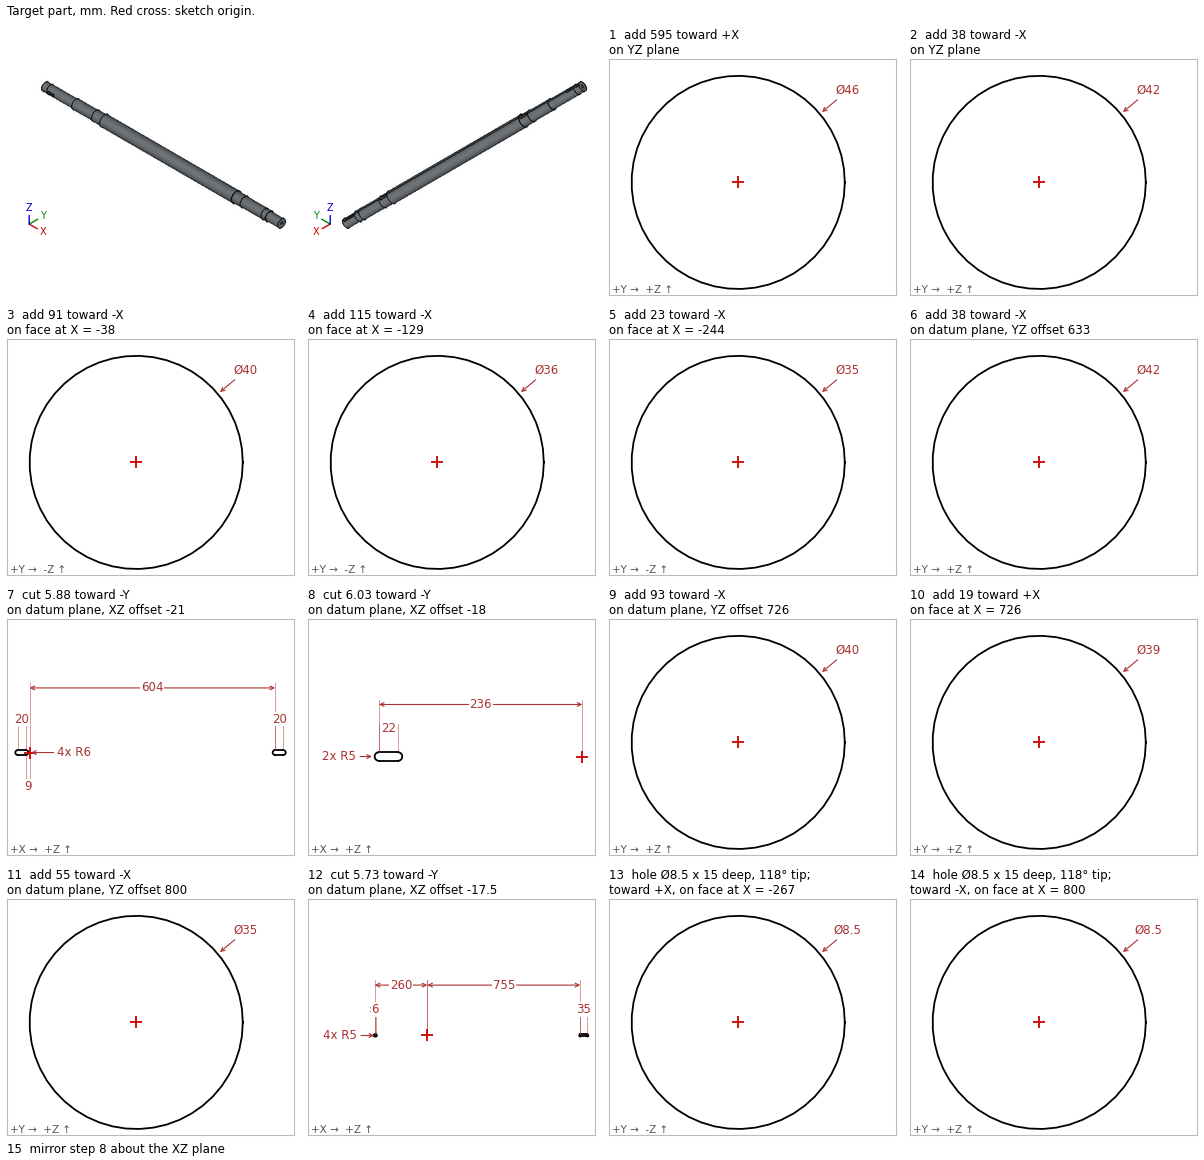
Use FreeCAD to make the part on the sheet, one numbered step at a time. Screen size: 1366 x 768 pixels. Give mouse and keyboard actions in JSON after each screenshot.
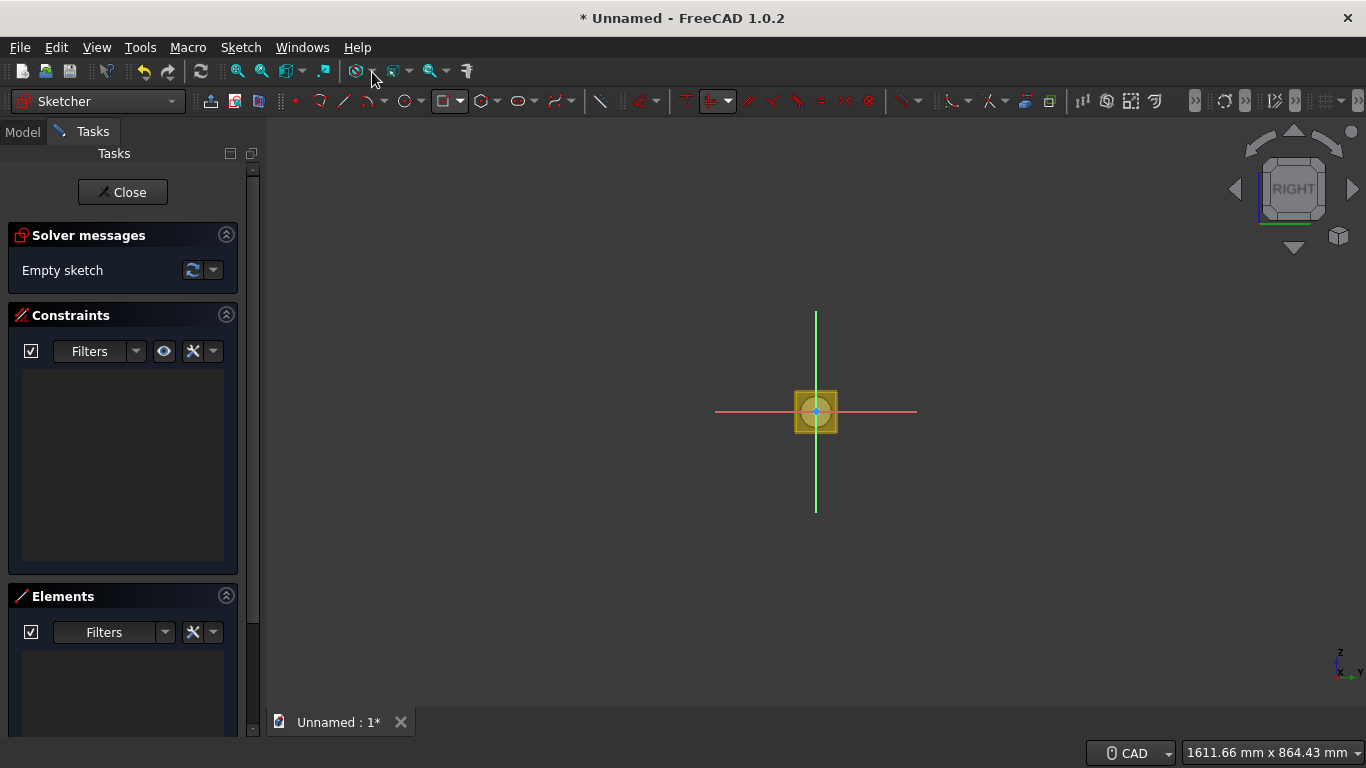
{"action": "scroll", "coordinate": [821, 412], "scroll_direction": "up", "scroll_amount": 13}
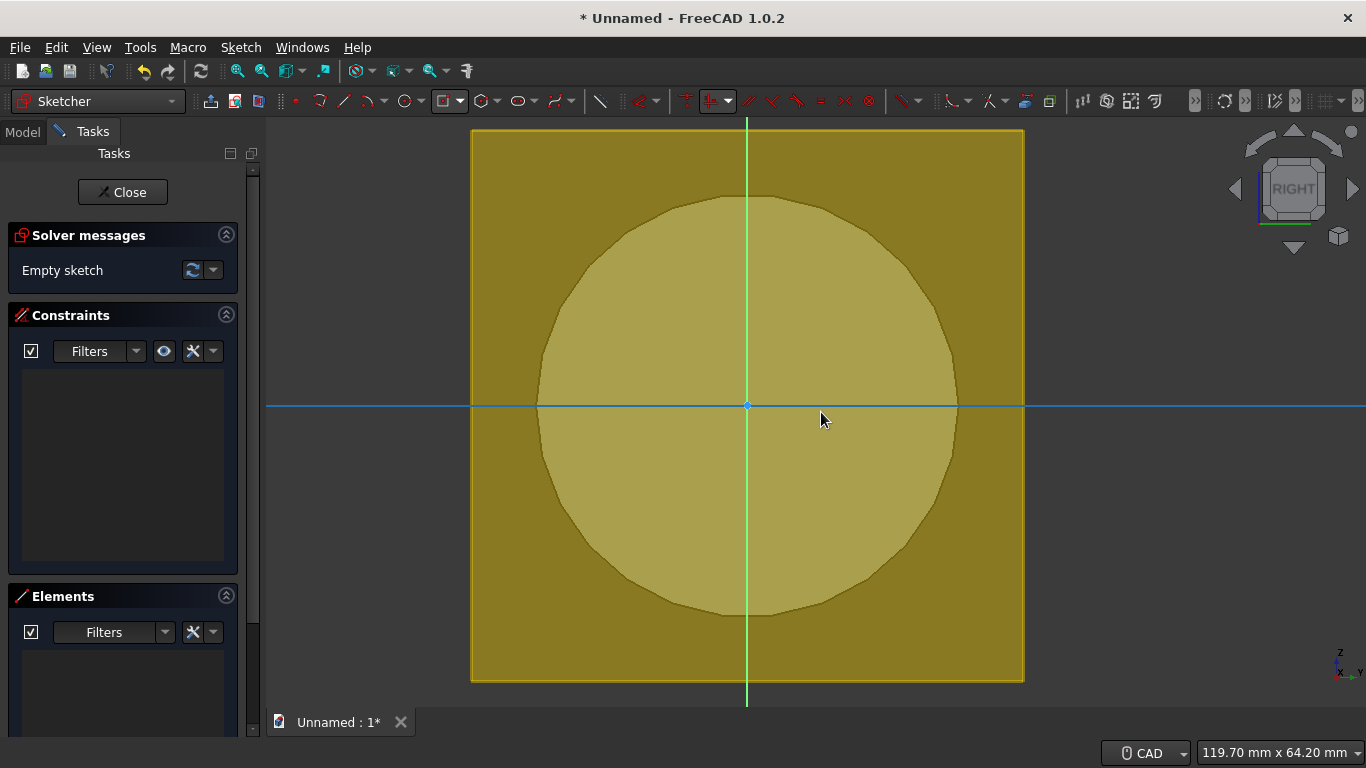
{"action": "key", "text": "g c"}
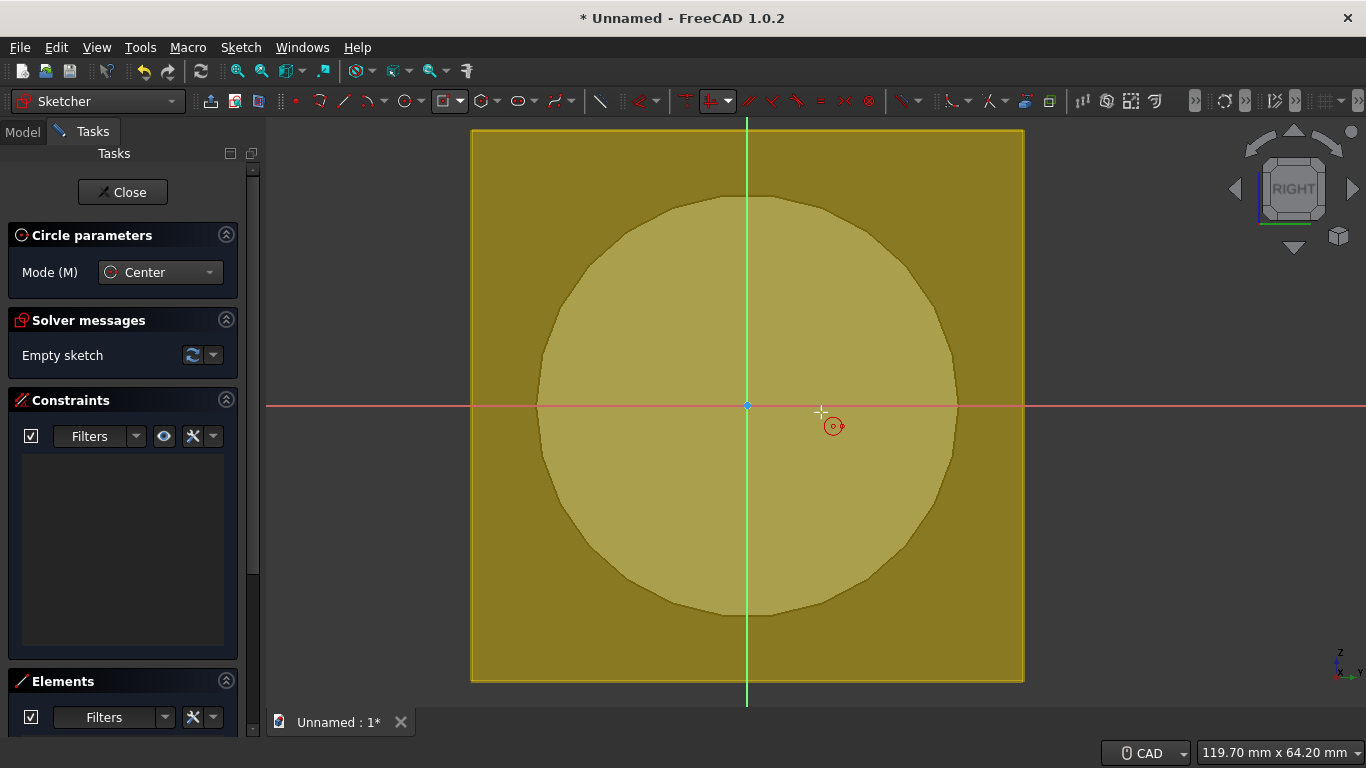
{"action": "left_click", "coordinate": [747, 406]}
{"action": "mouse_move", "coordinate": [884, 269]}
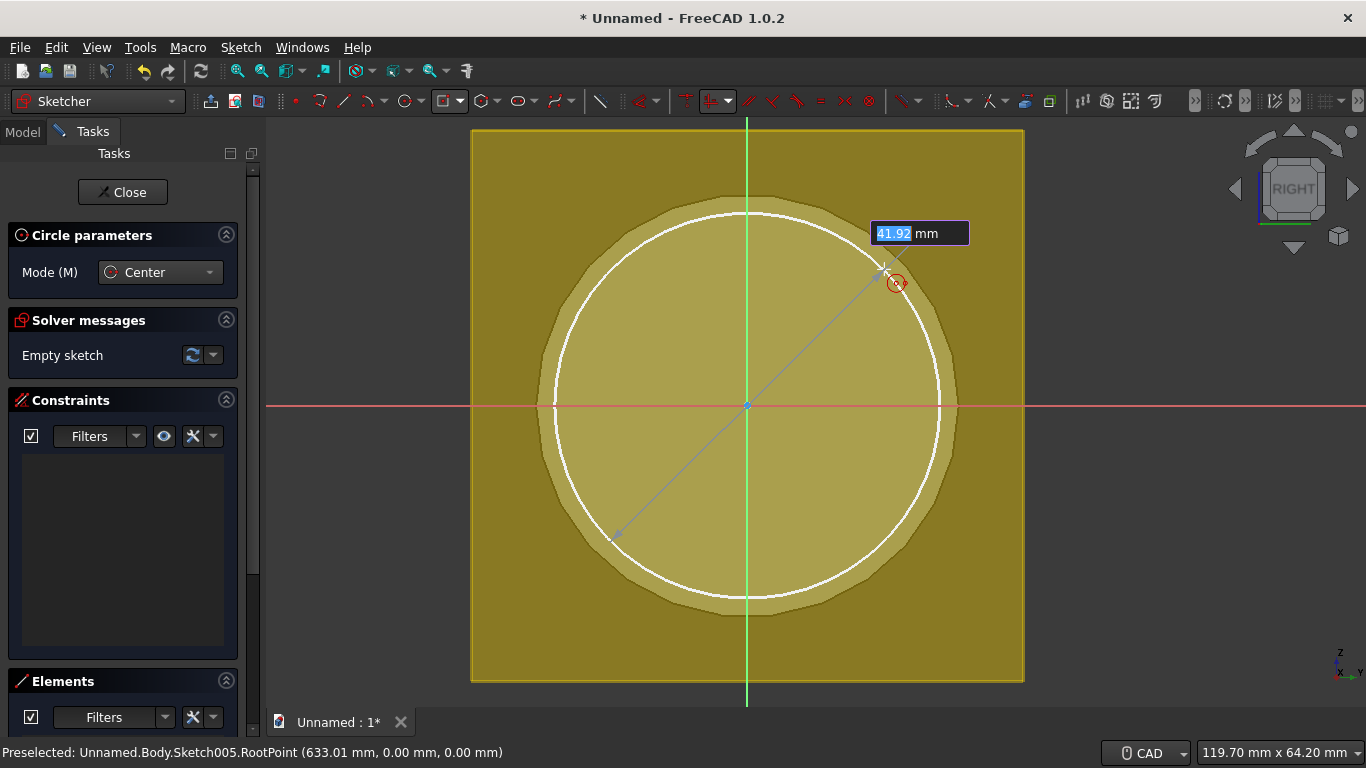
{"action": "type", "text": "42"}
{"action": "key", "text": "Return"}
{"action": "key", "text": "Escape"}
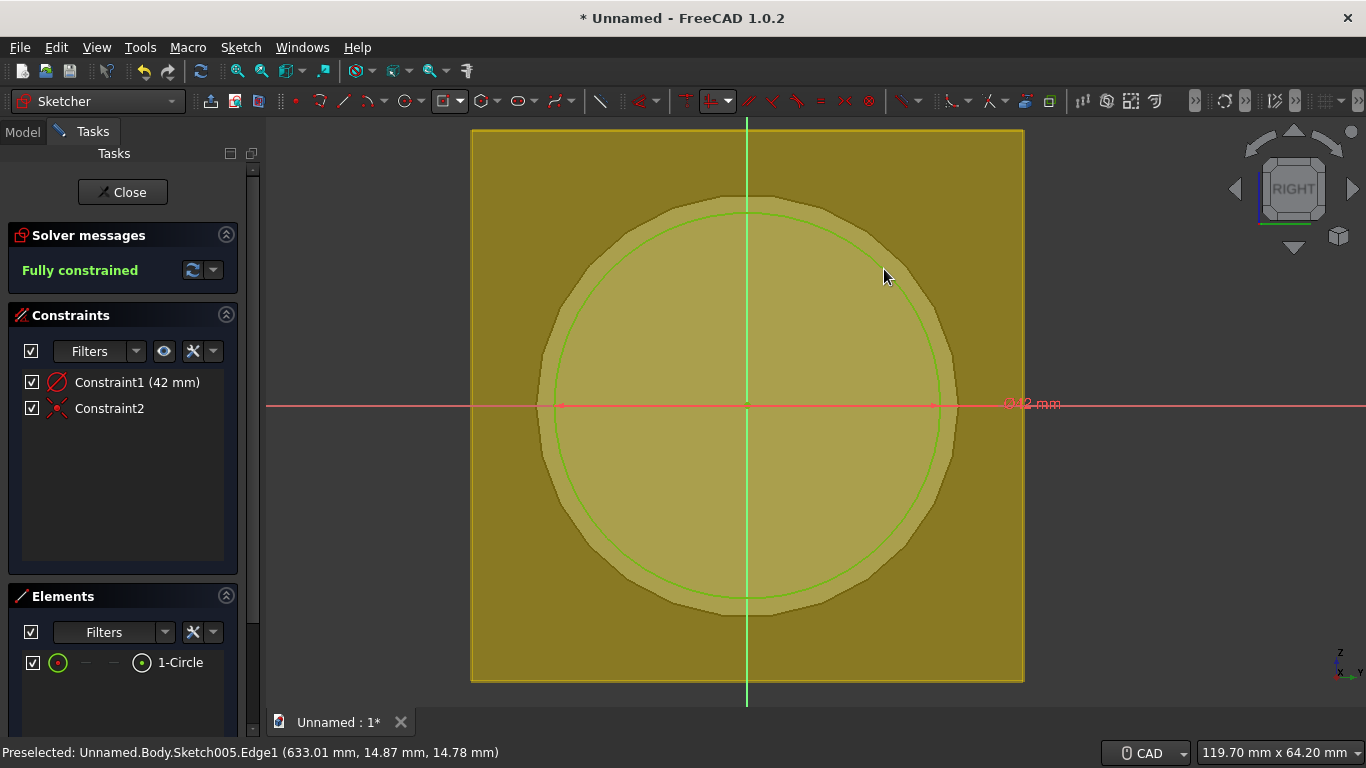
{"action": "left_click", "coordinate": [123, 192]}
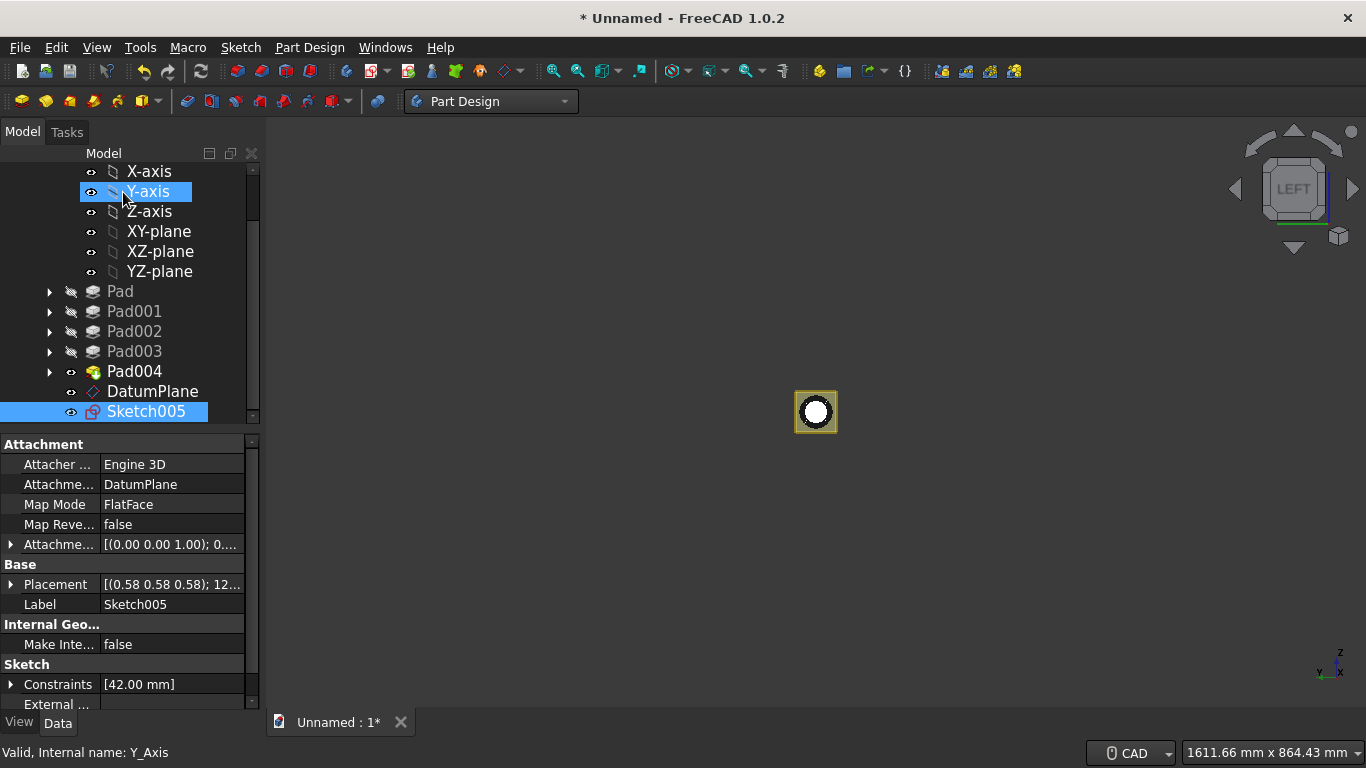
{"action": "left_click", "coordinate": [22, 102]}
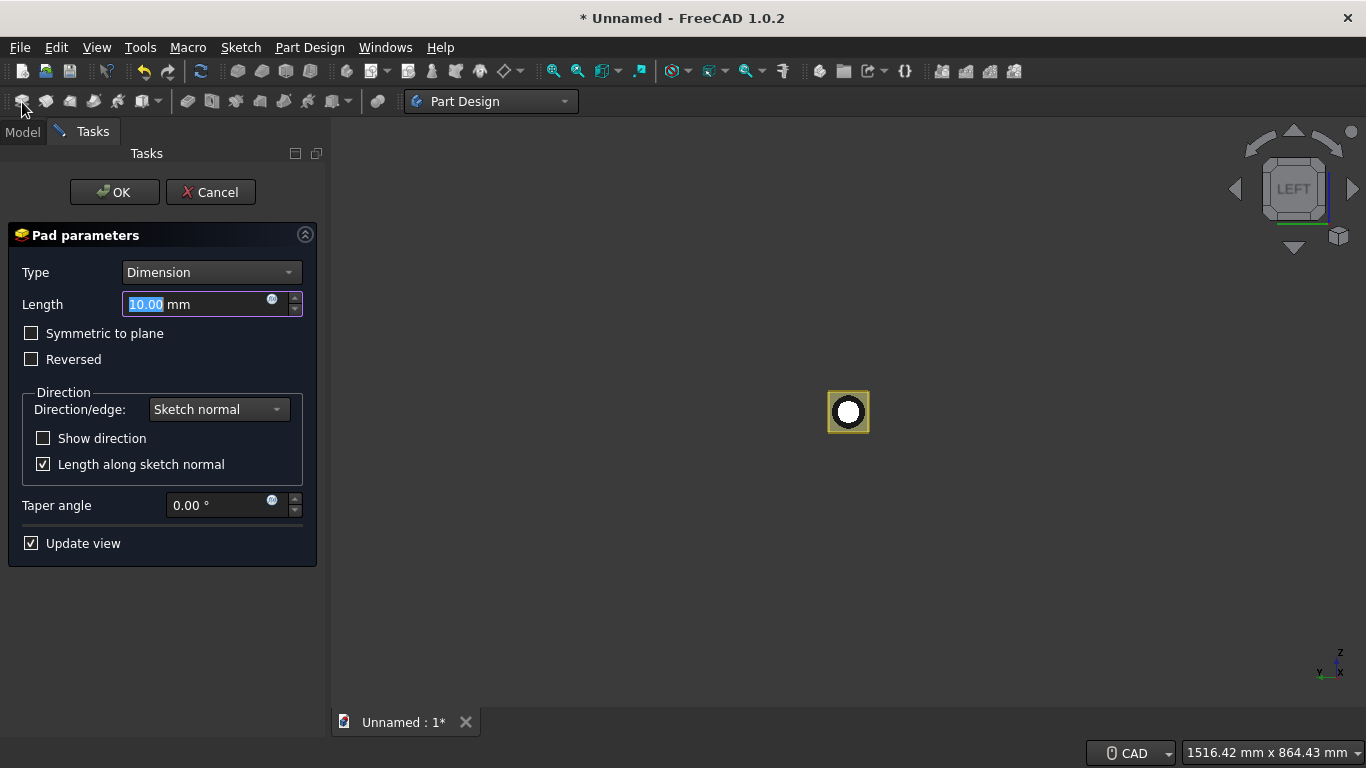
{"action": "type", "text": "38"}
{"action": "key", "text": "Tab"}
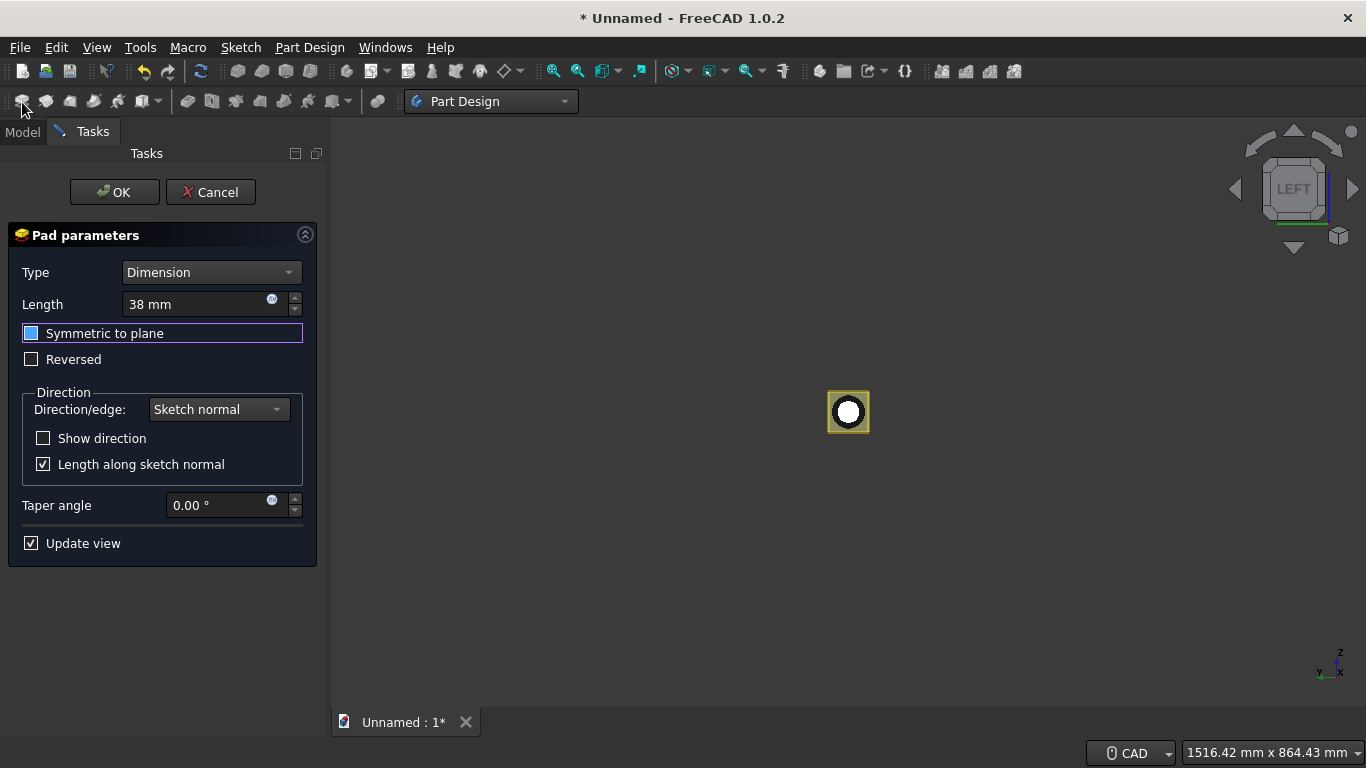
{"action": "left_click", "coordinate": [30, 359]}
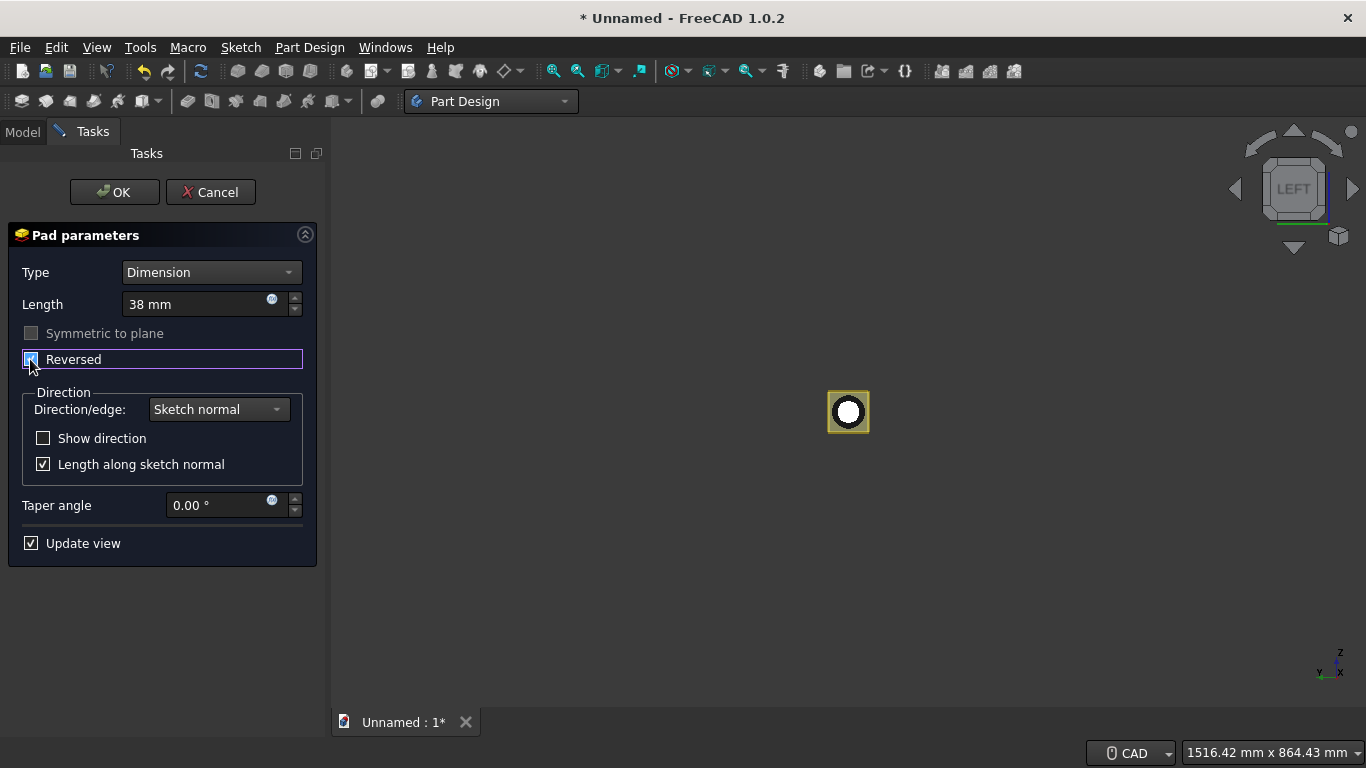
{"action": "left_click", "coordinate": [115, 192]}